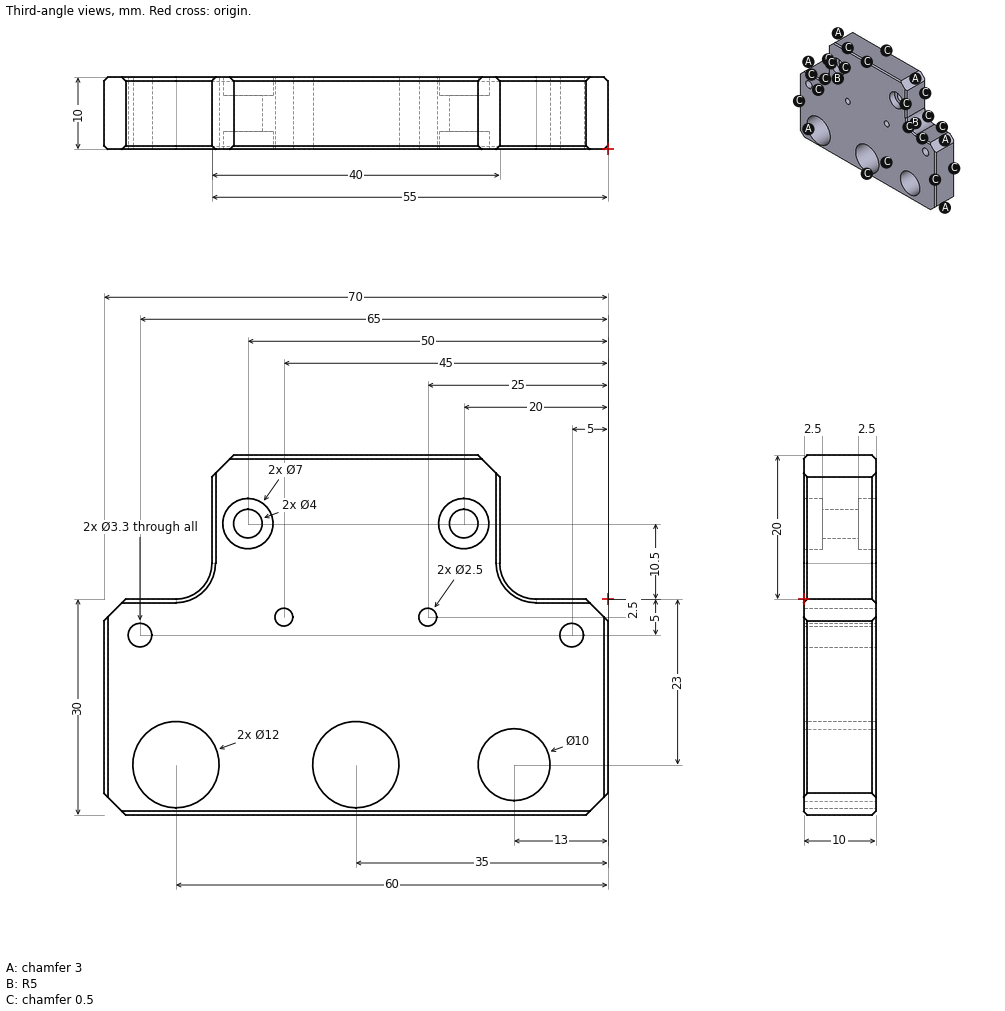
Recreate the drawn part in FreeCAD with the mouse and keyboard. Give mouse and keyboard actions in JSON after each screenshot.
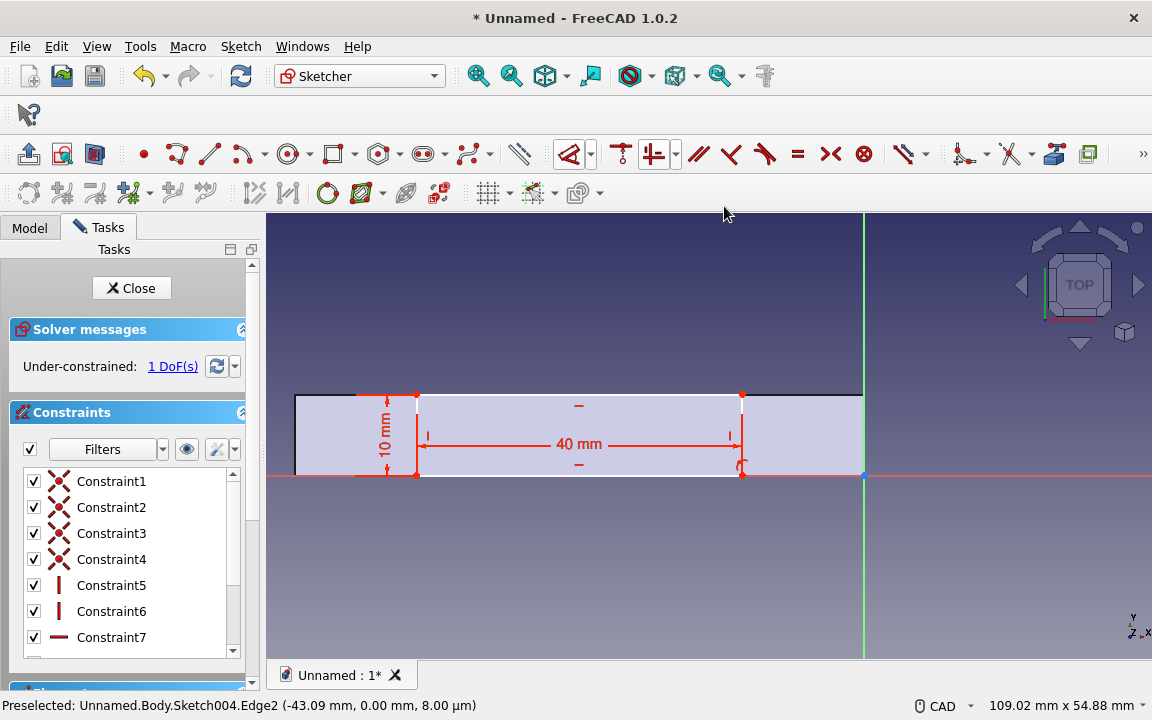
{"action": "left_click", "coordinate": [417, 395]}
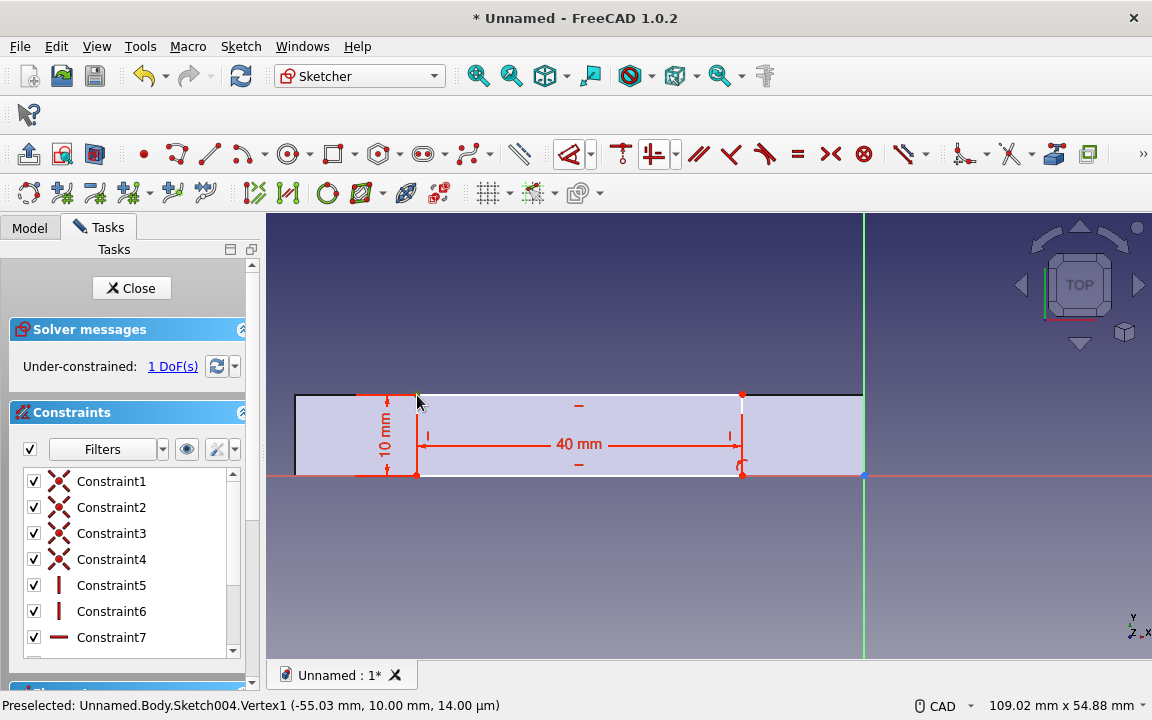
{"action": "key", "text": "l"}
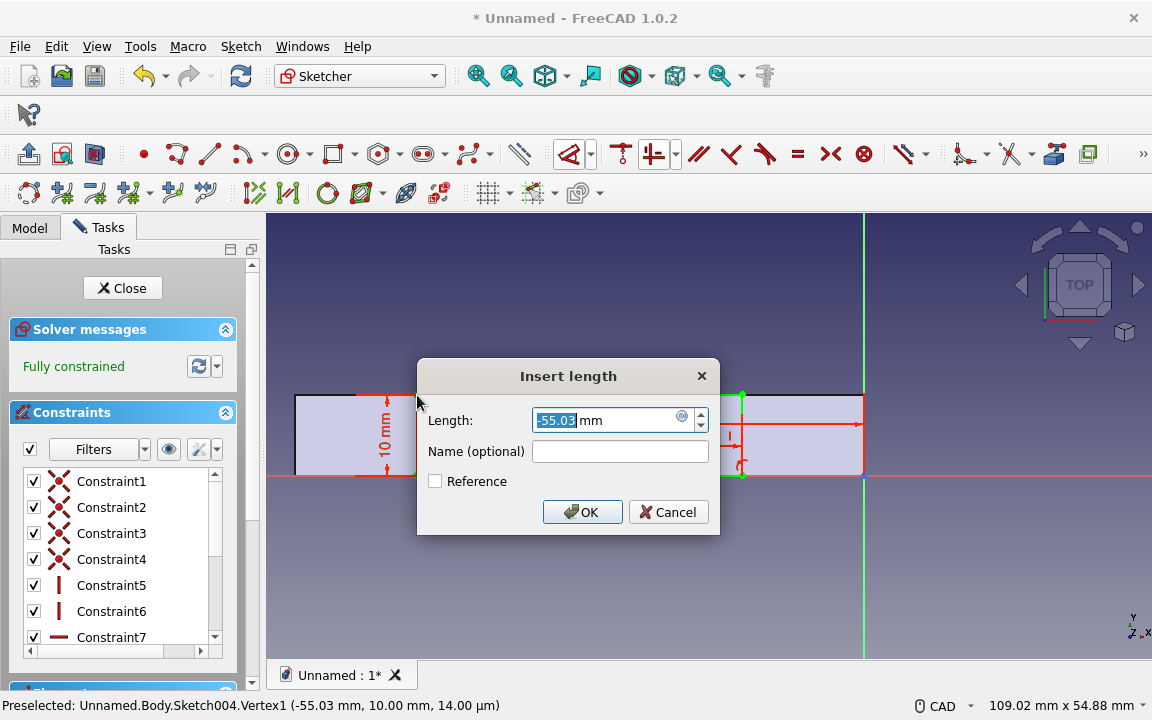
{"action": "type", "text": "-55"}
{"action": "key", "text": "Return"}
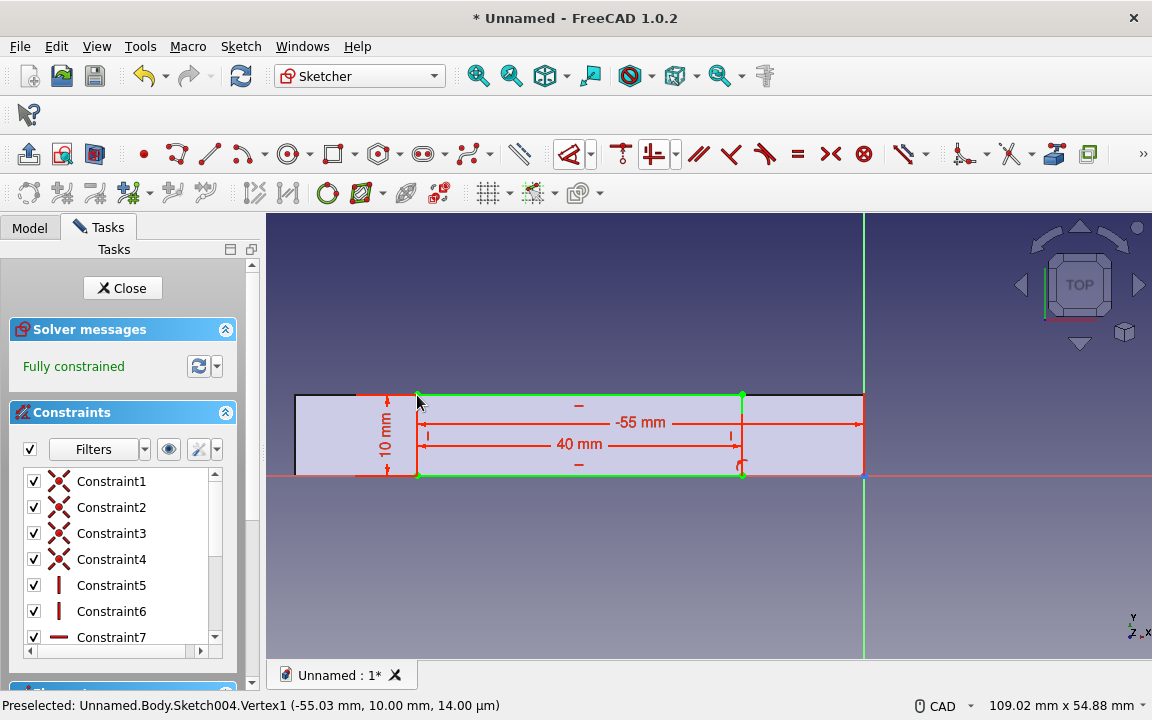
{"action": "left_click", "coordinate": [123, 288]}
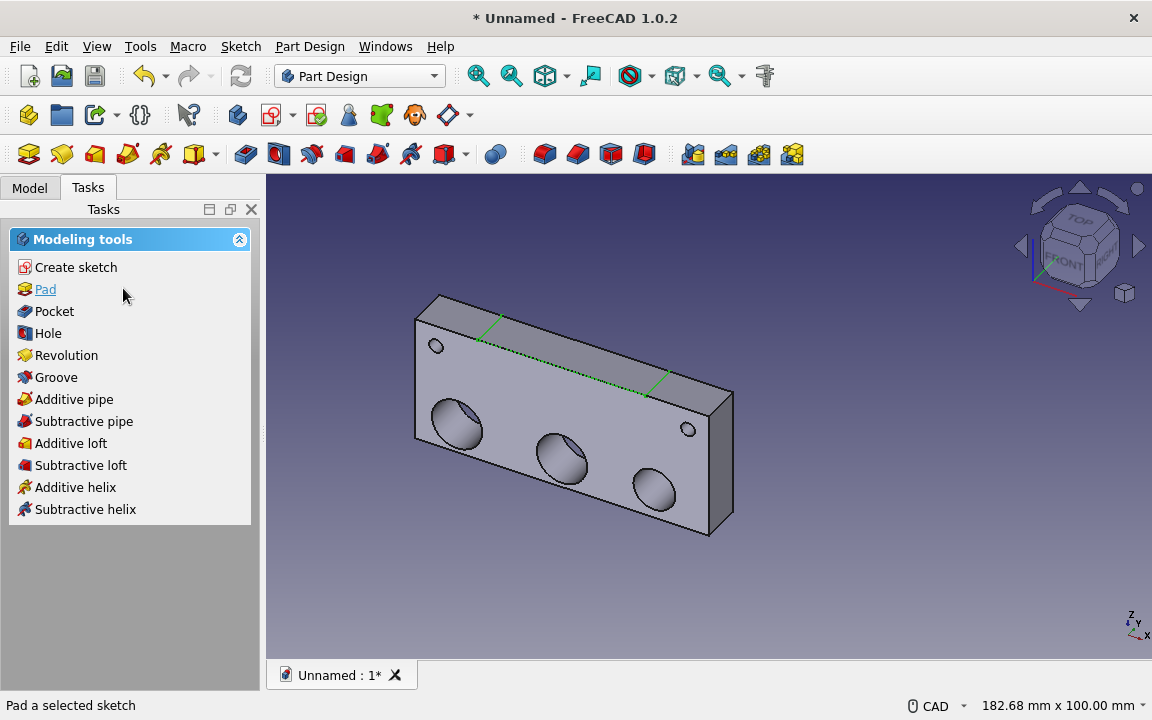
{"action": "left_click", "coordinate": [29, 154]}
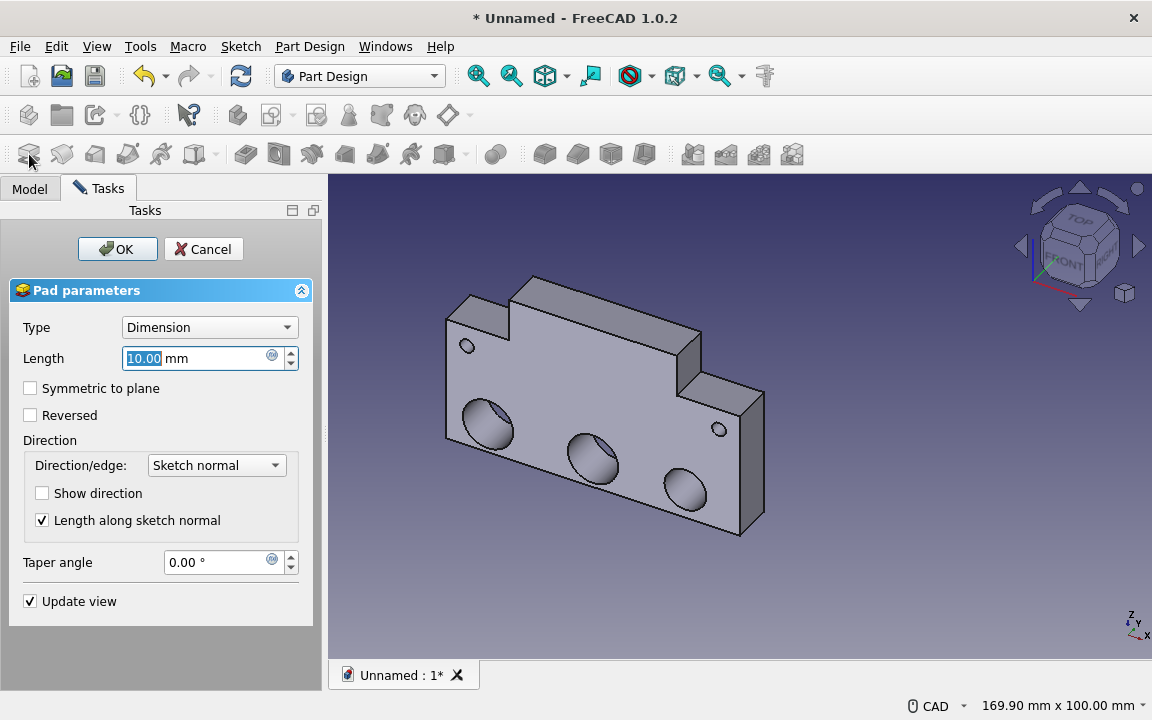
{"action": "type", "text": "20"}
{"action": "key", "text": "Tab"}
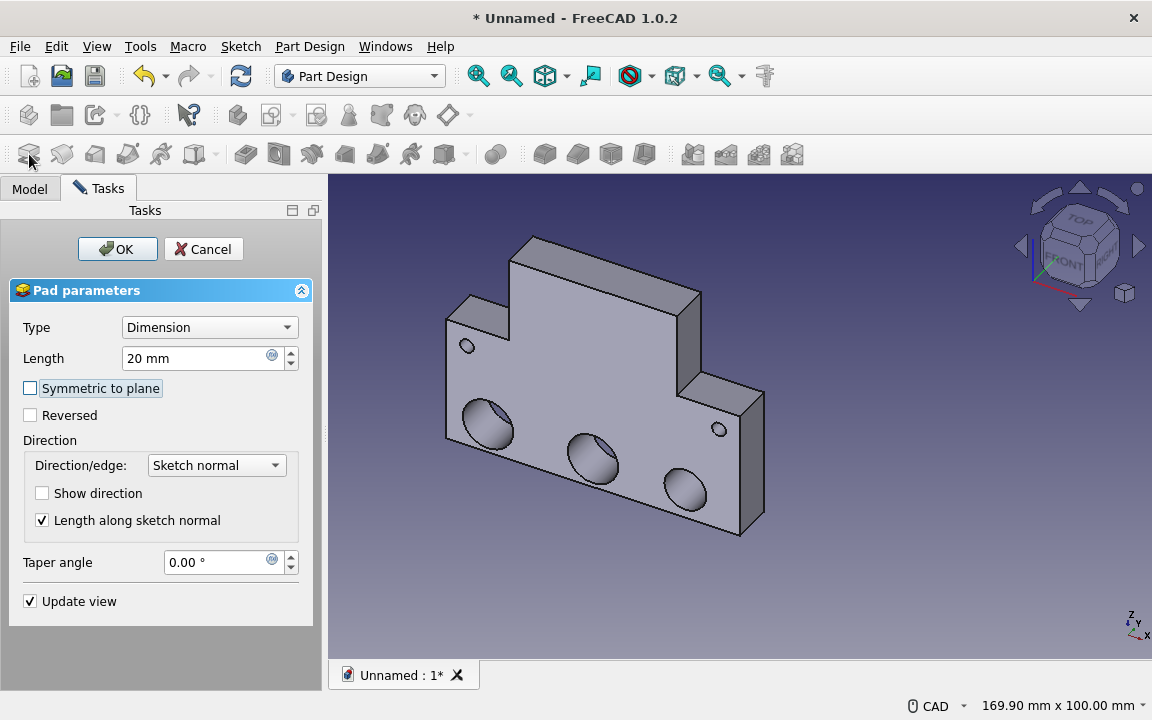
{"action": "left_click", "coordinate": [118, 249]}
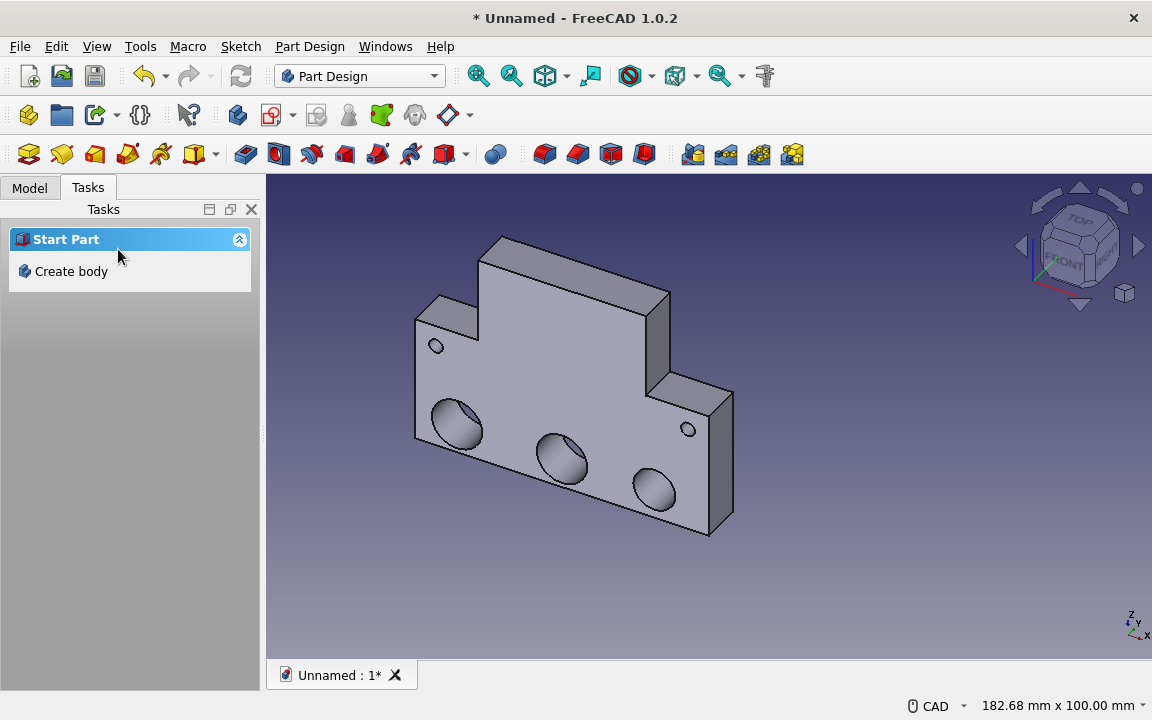
{"action": "key", "text": "4"}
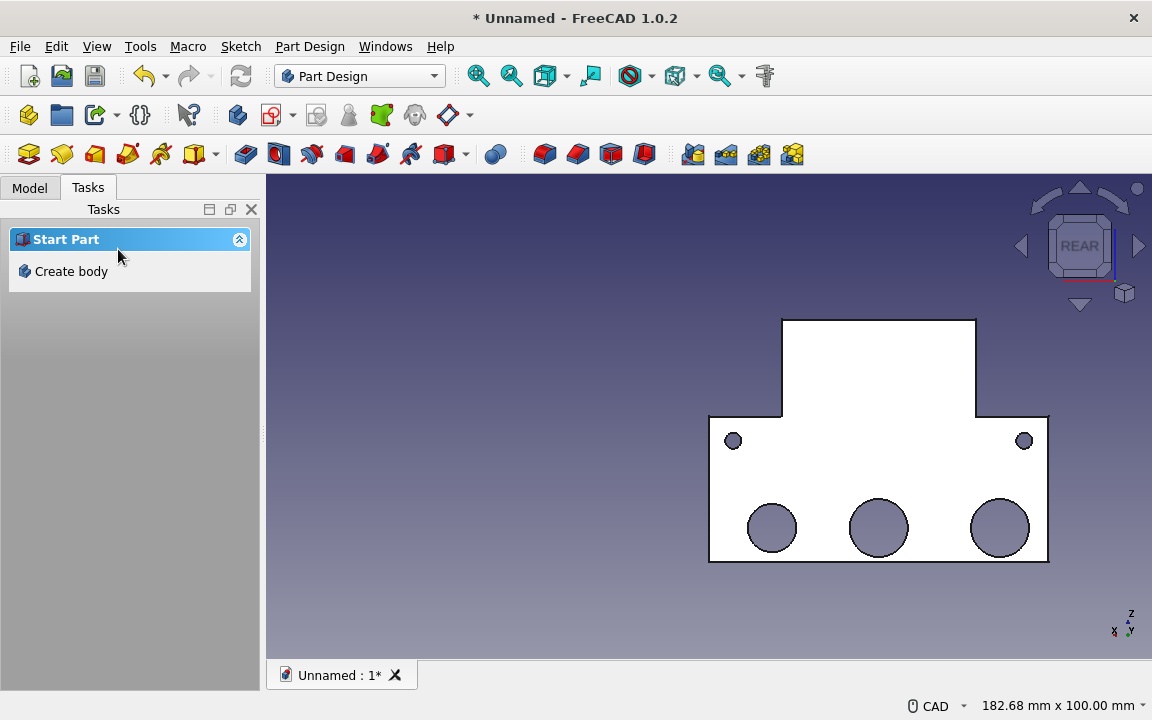
{"action": "left_click", "coordinate": [879, 405]}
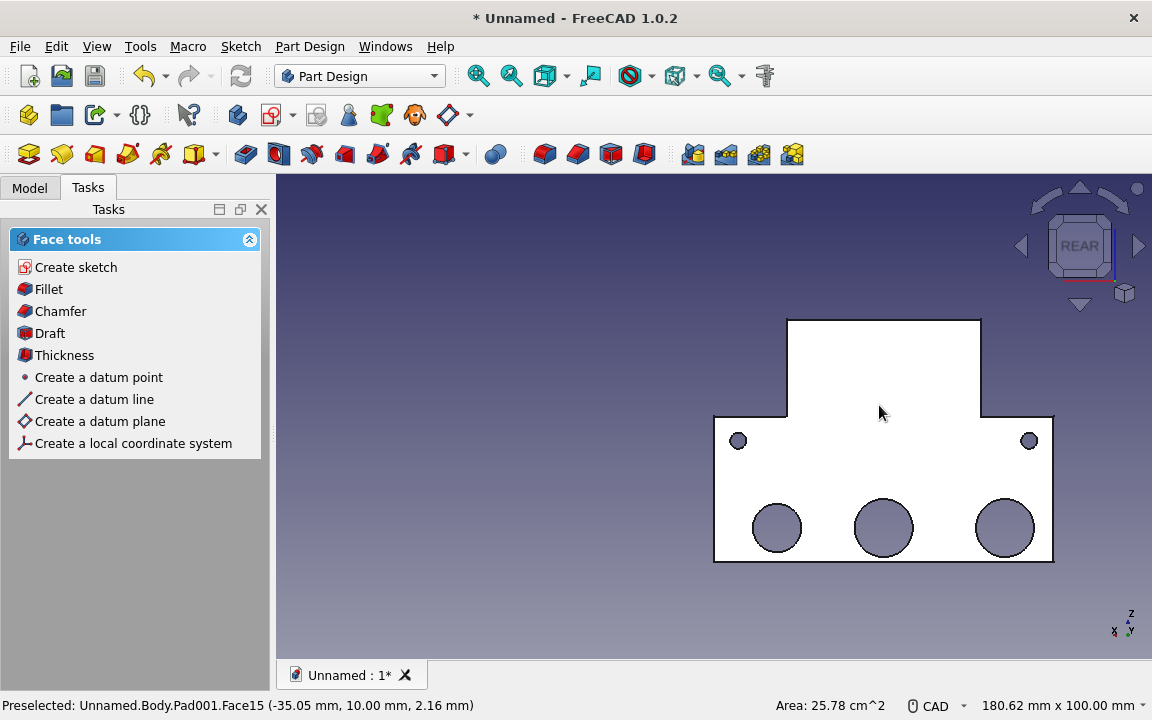
{"action": "left_click", "coordinate": [270, 116]}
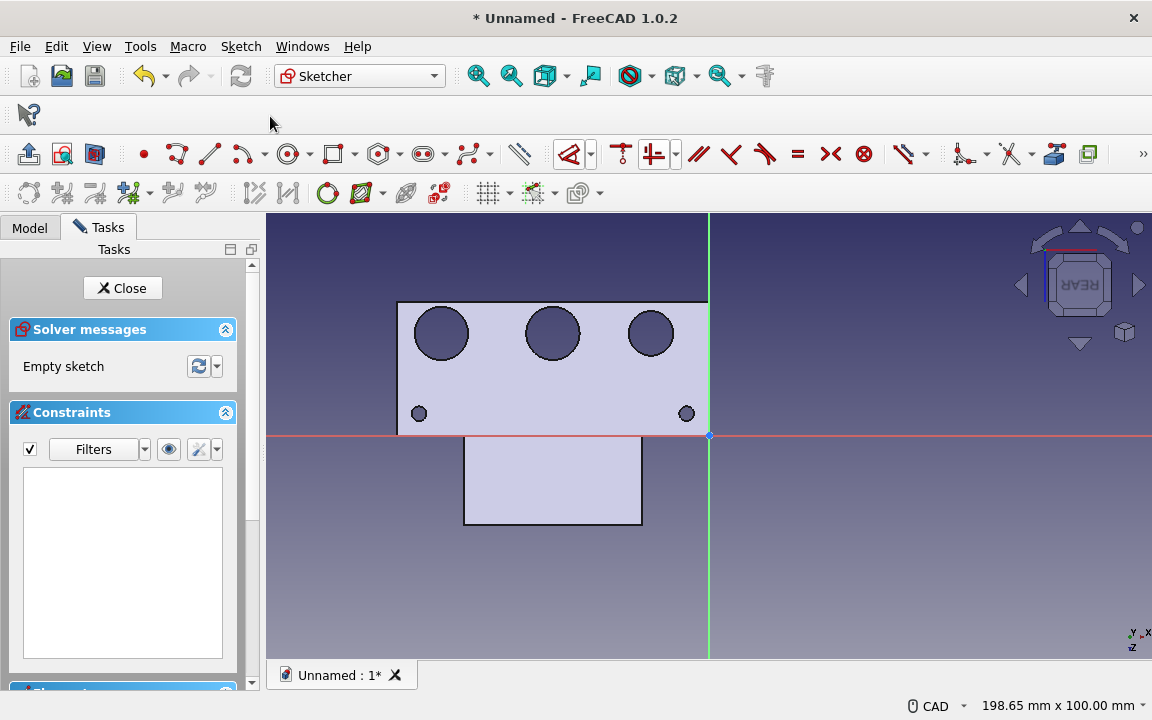
{"action": "scroll", "coordinate": [554, 487], "scroll_direction": "up", "scroll_amount": 4}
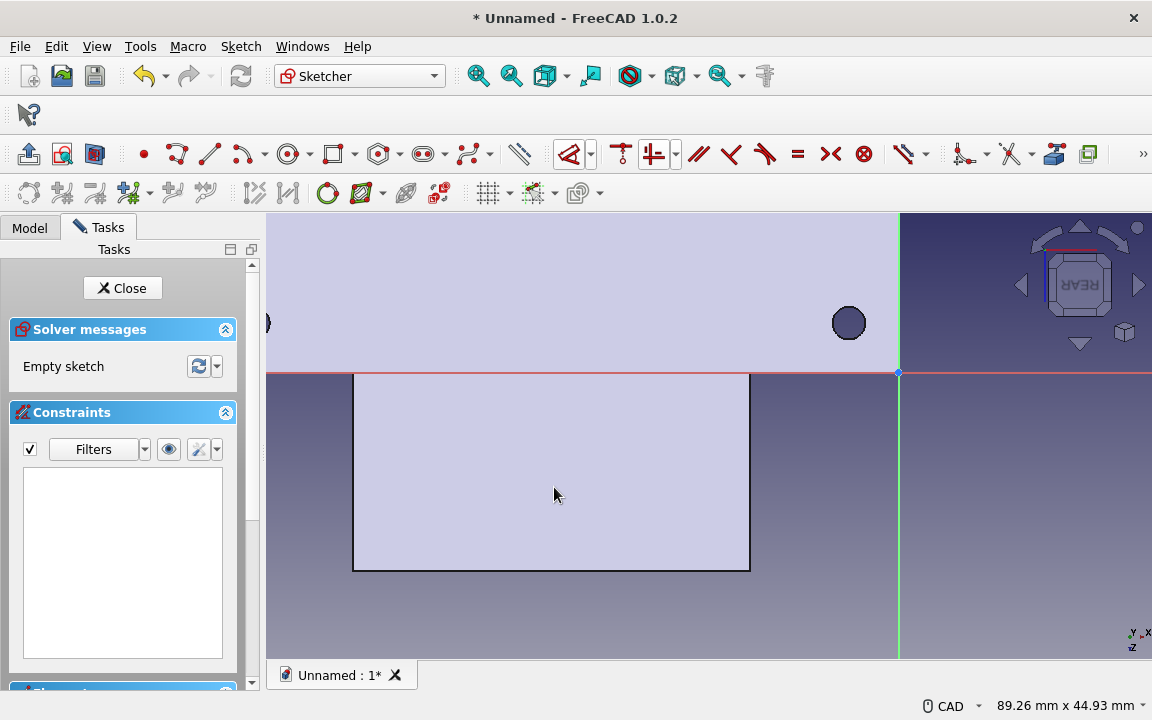
{"action": "left_click", "coordinate": [288, 154]}